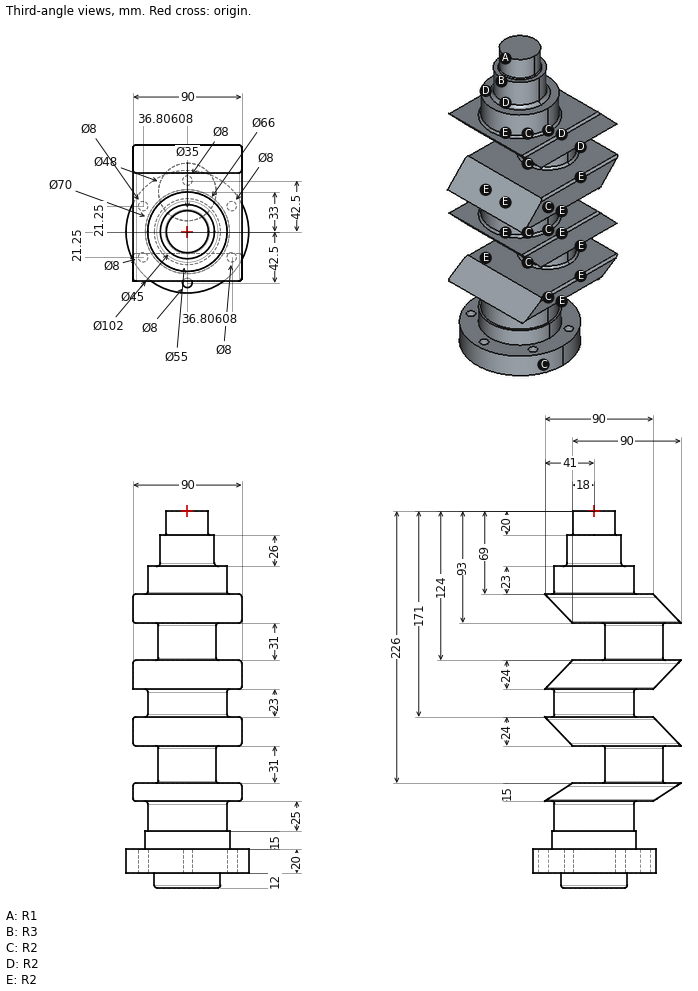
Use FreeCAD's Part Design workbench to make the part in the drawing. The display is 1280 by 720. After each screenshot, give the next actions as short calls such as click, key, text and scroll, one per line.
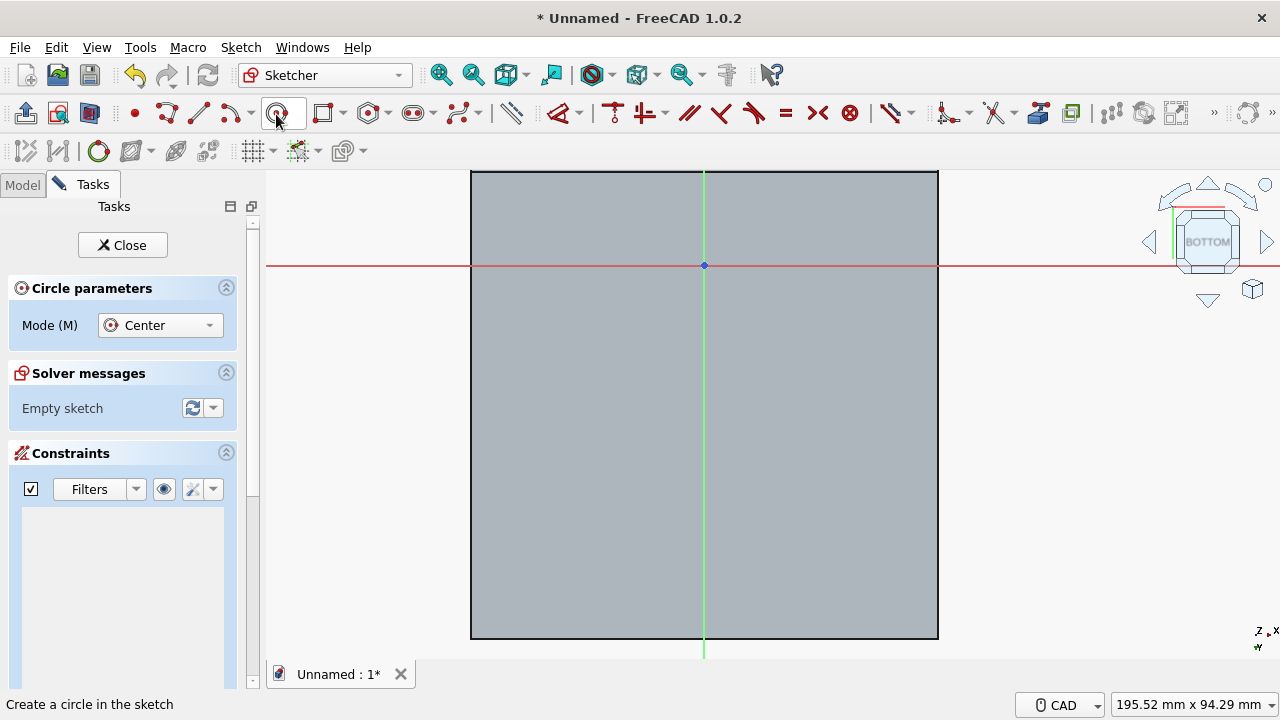
click(704, 437)
move(792, 349)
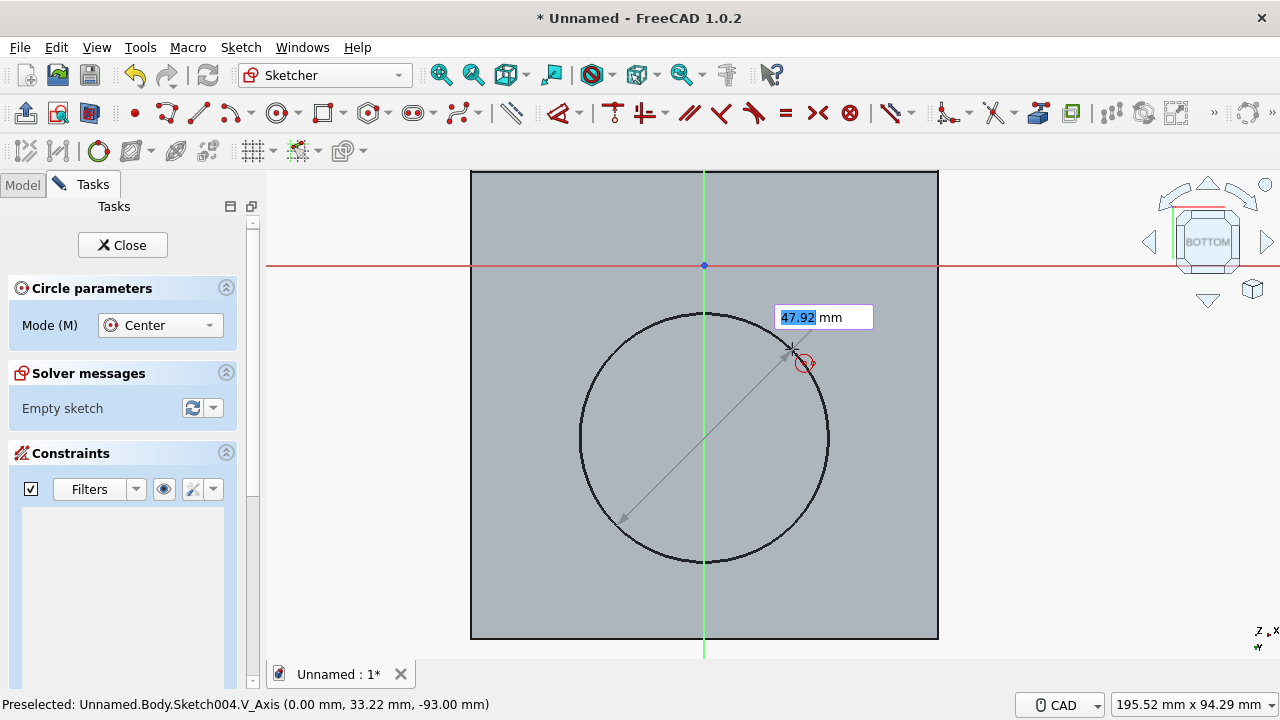
text(48)
key(Return)
key(Escape)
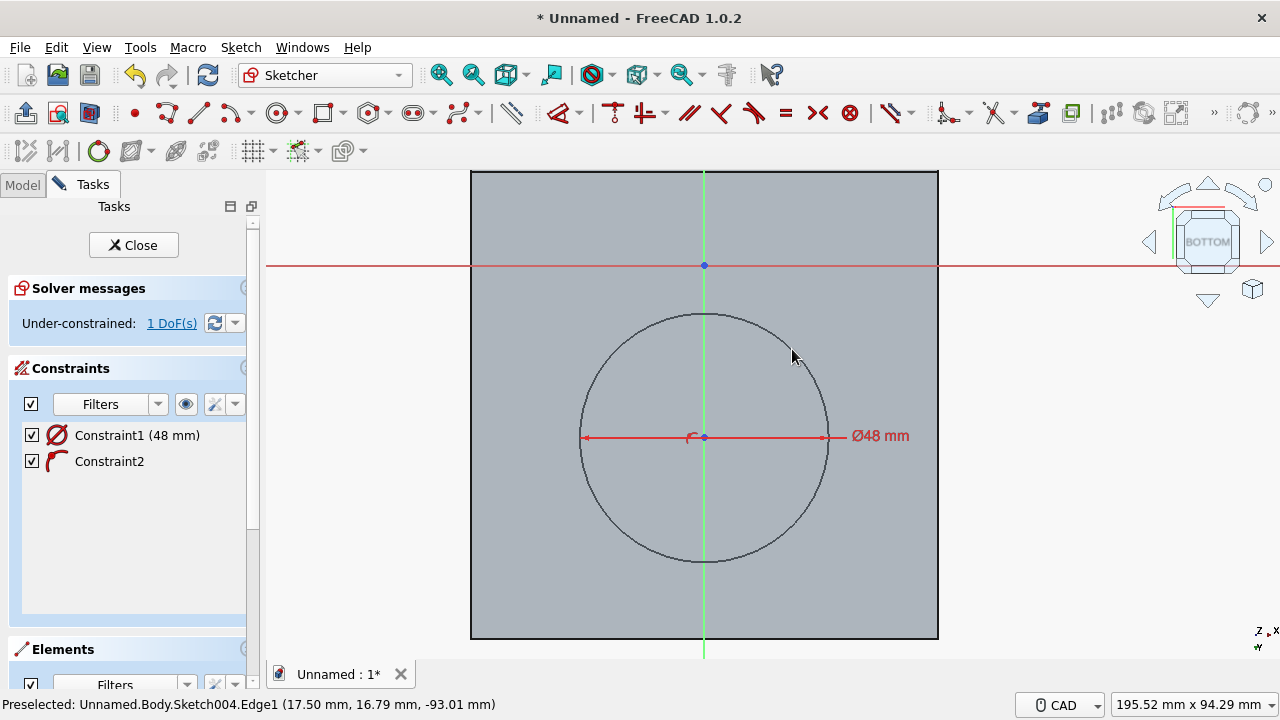
click(558, 114)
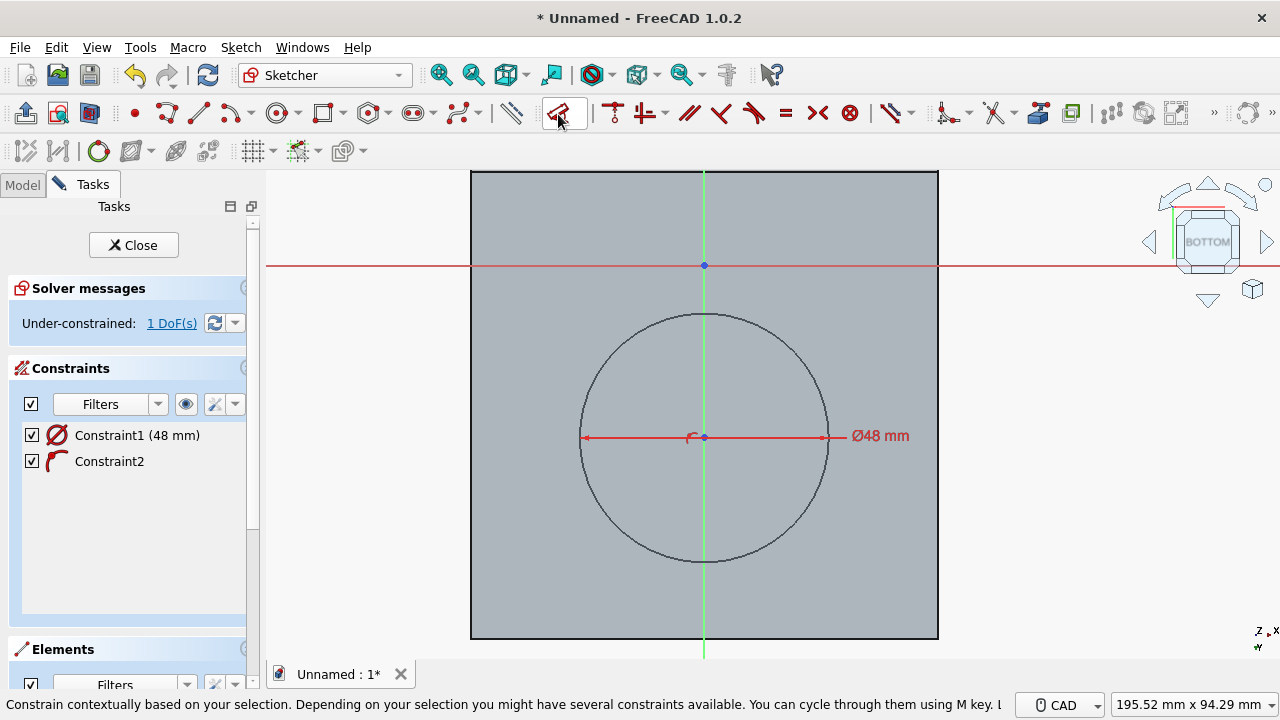
click(704, 438)
click(738, 352)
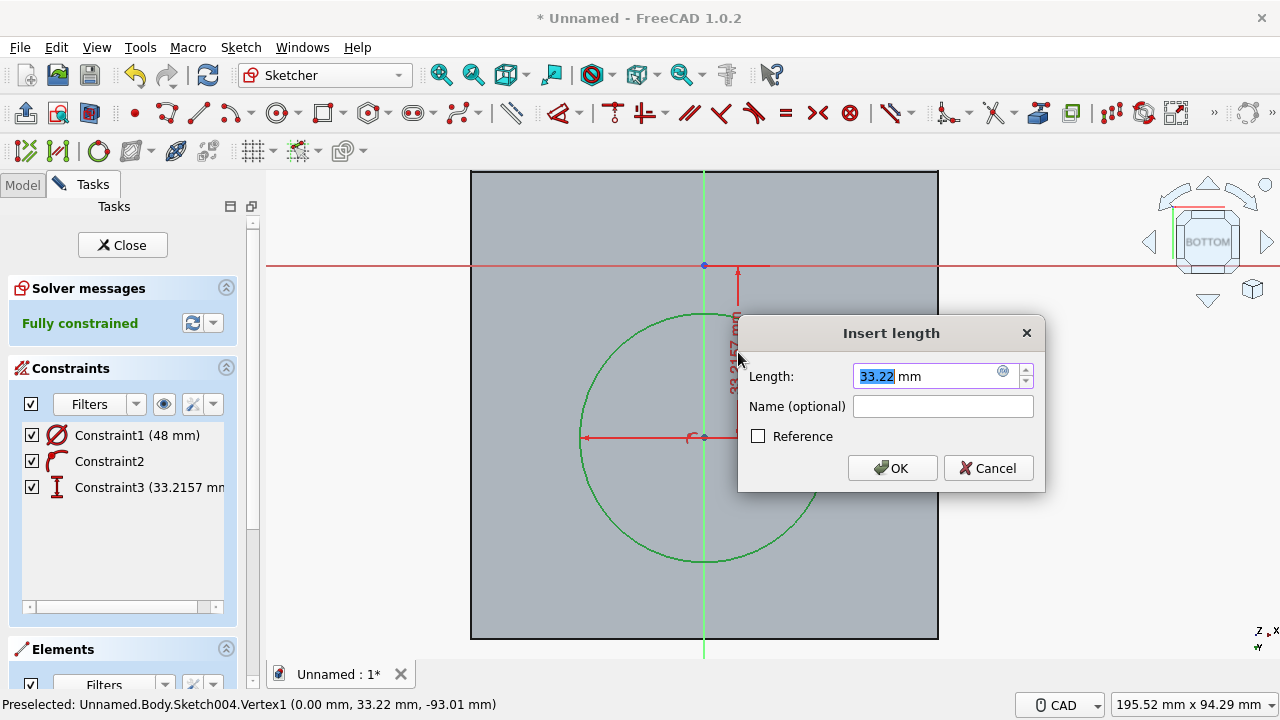
text(33)
key(Return)
key(Escape)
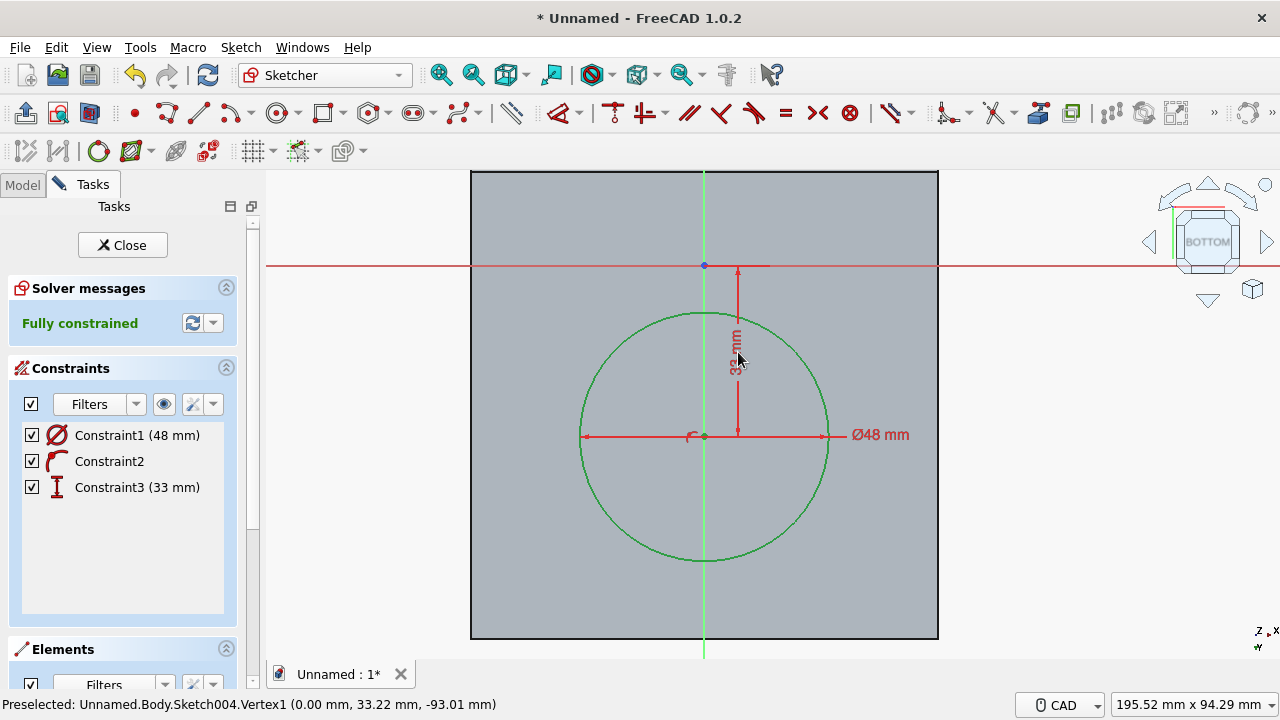
click(123, 245)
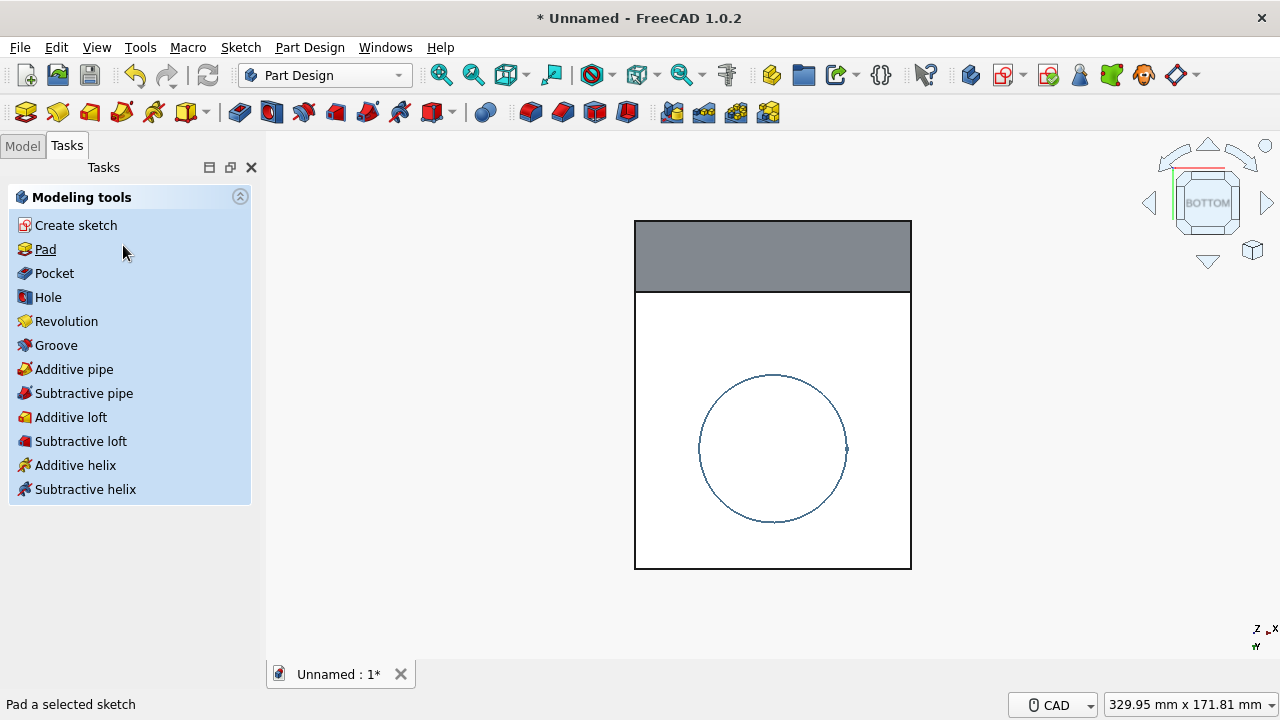
click(26, 112)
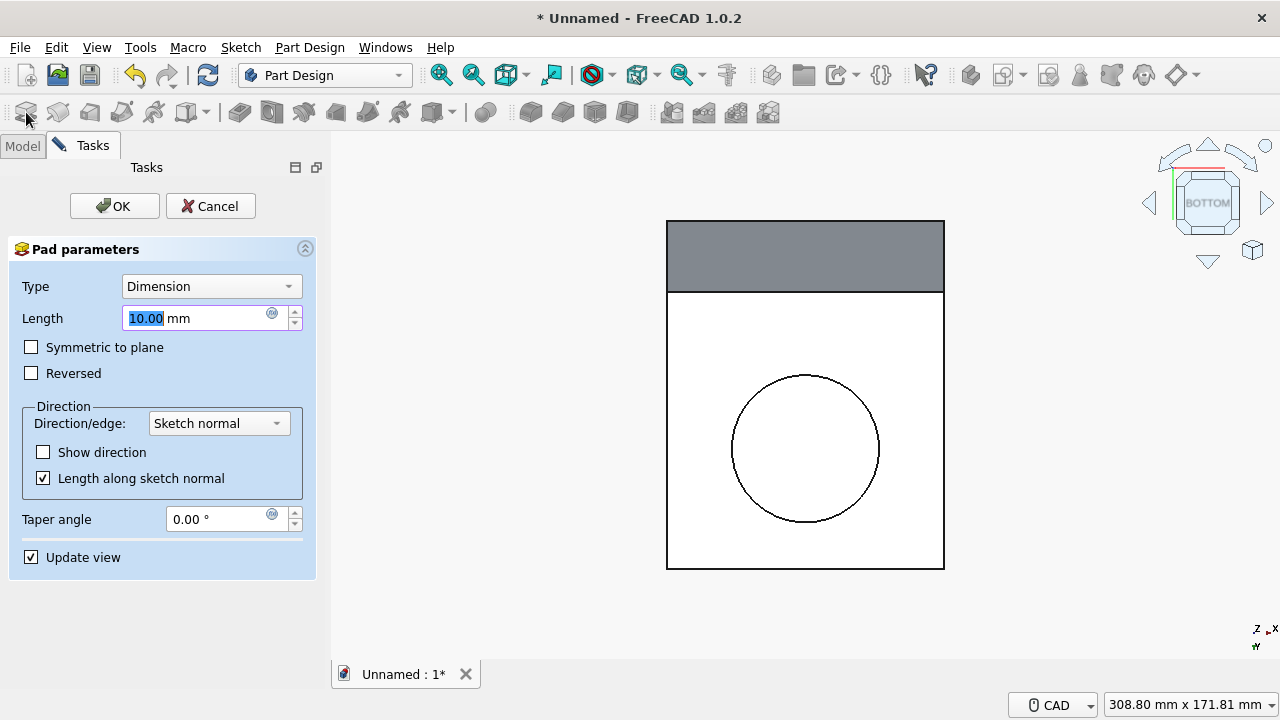
text(31)
key(Tab)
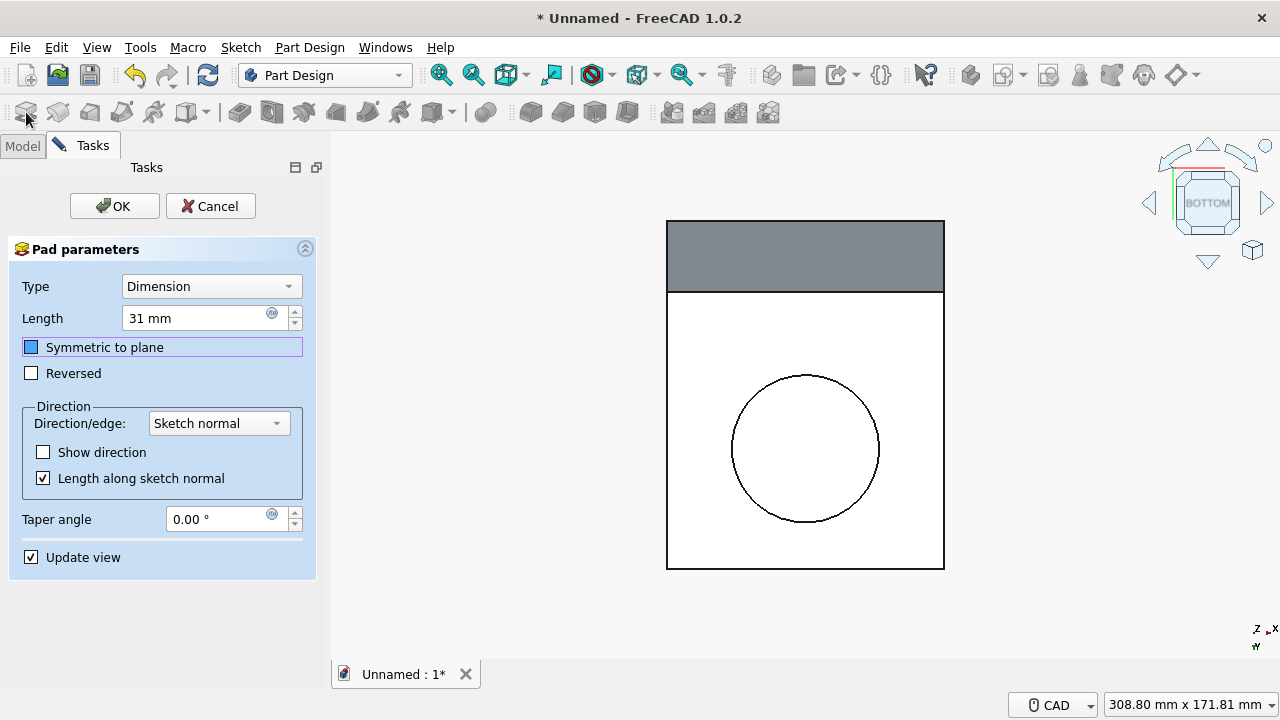
click(115, 206)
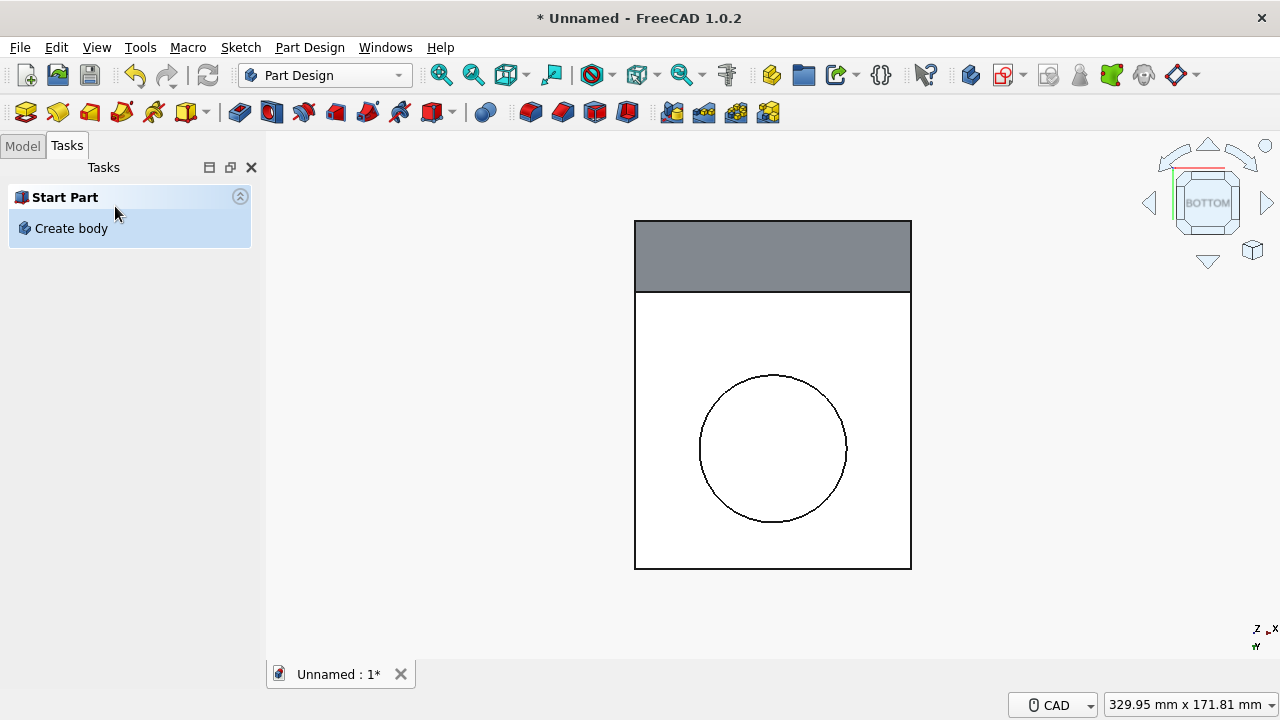
click(1004, 76)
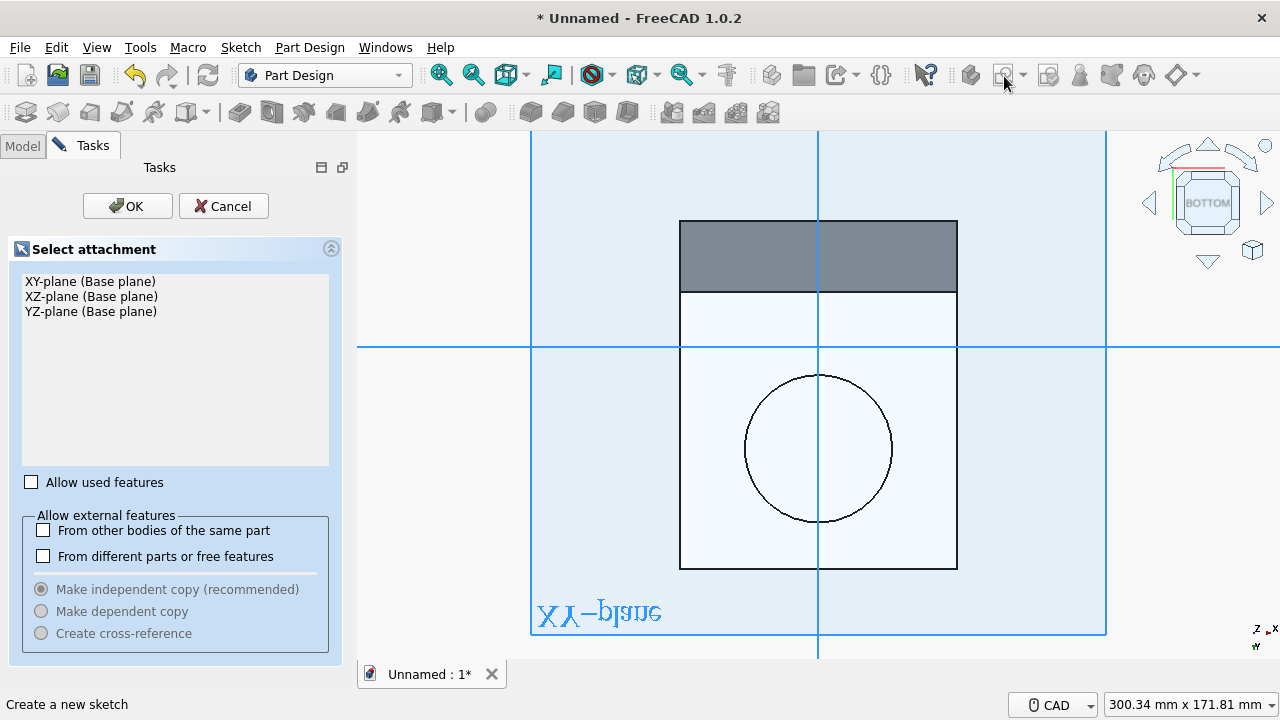
click(82, 312)